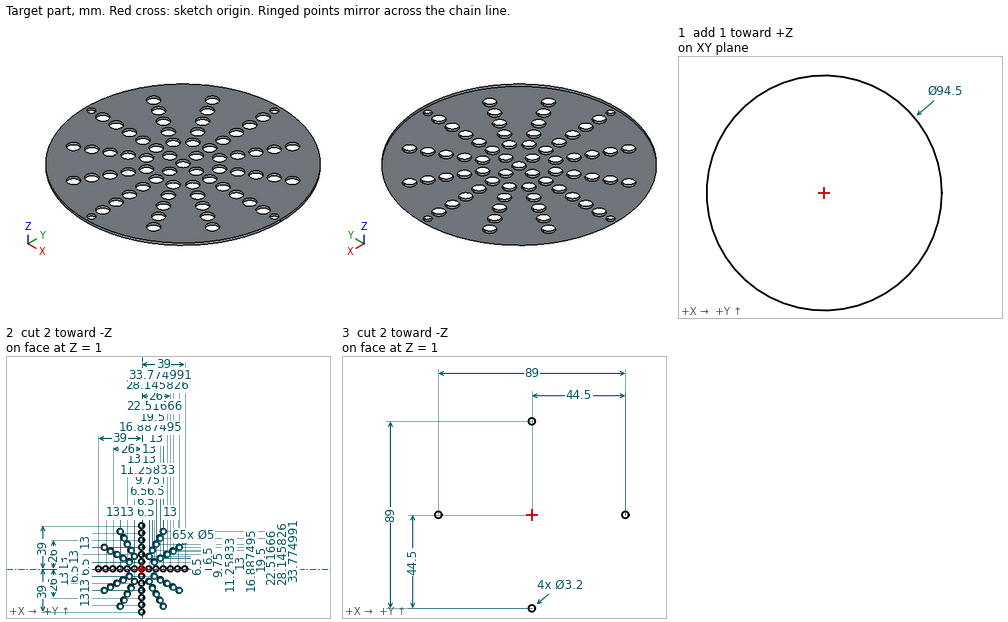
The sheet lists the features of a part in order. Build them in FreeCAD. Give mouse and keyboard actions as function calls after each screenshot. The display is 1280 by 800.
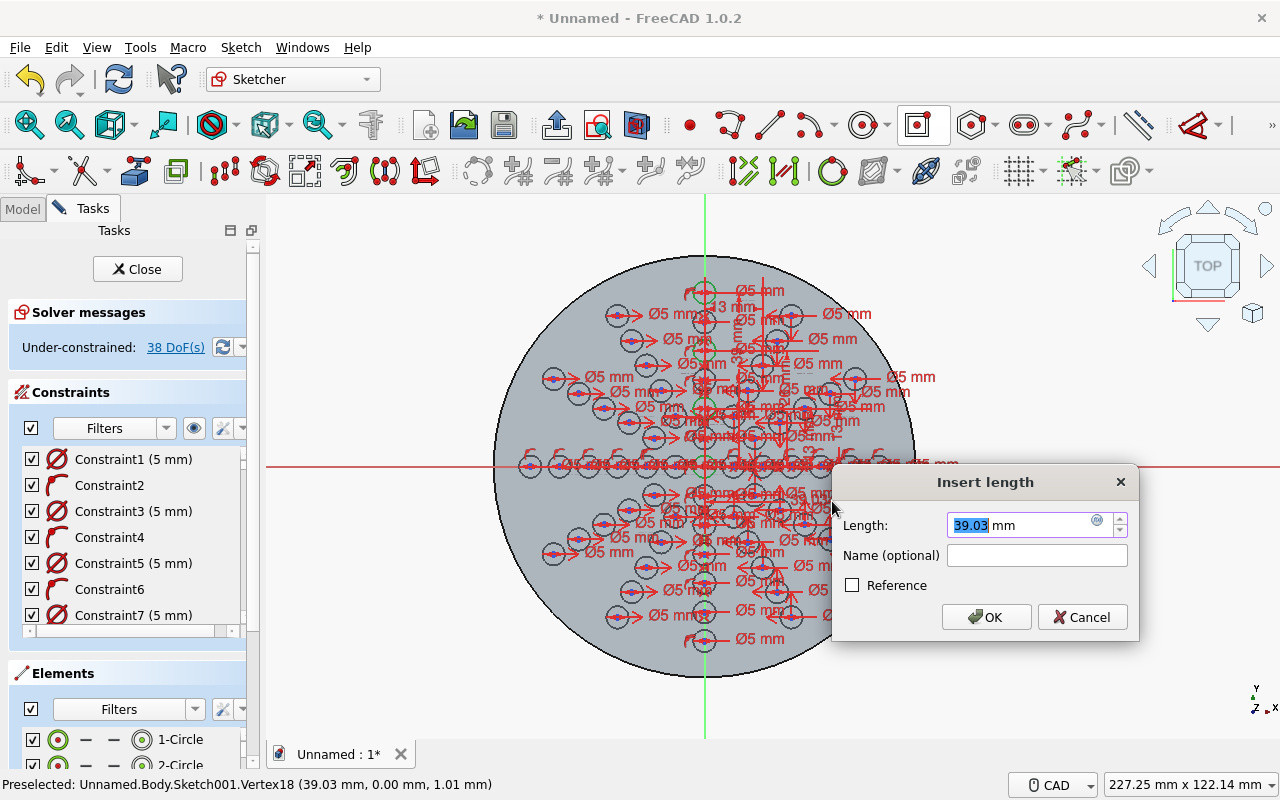
text(39)
key(Return)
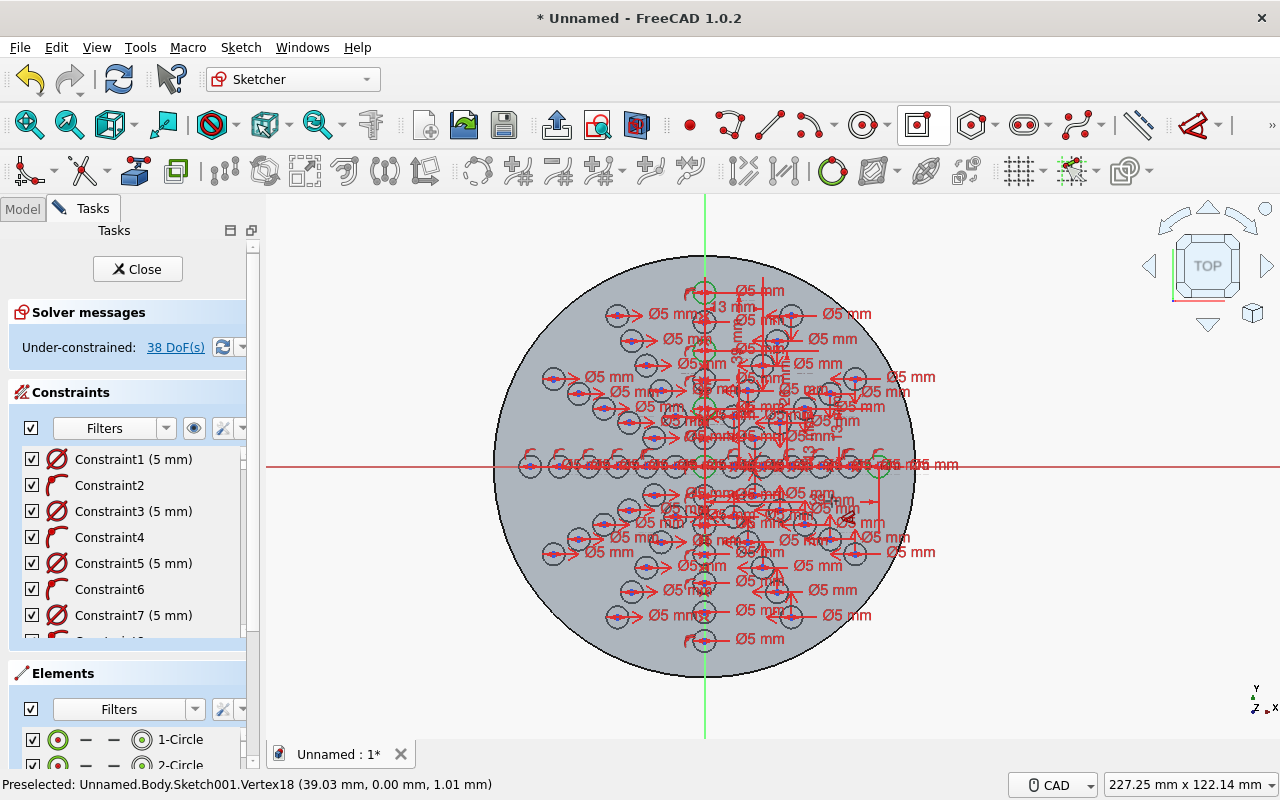
click(821, 467)
click(789, 549)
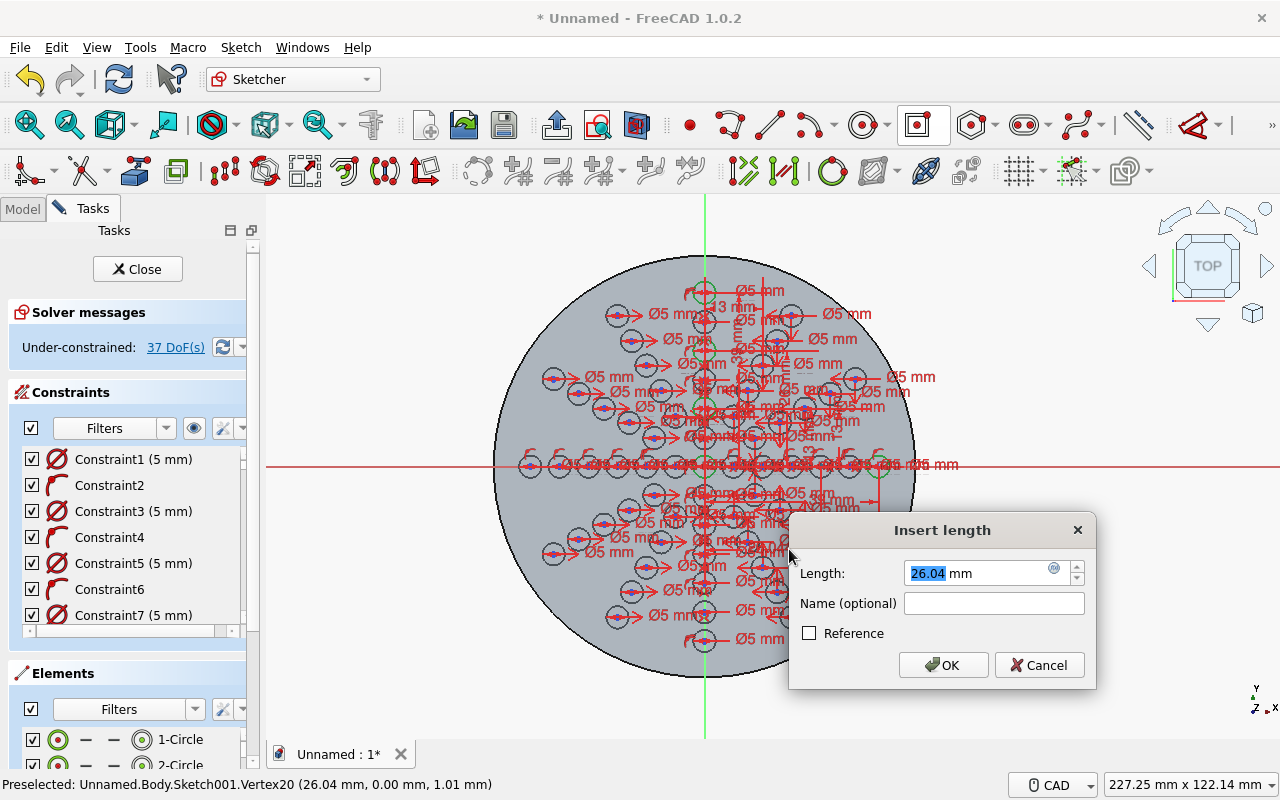
text(26)
key(Return)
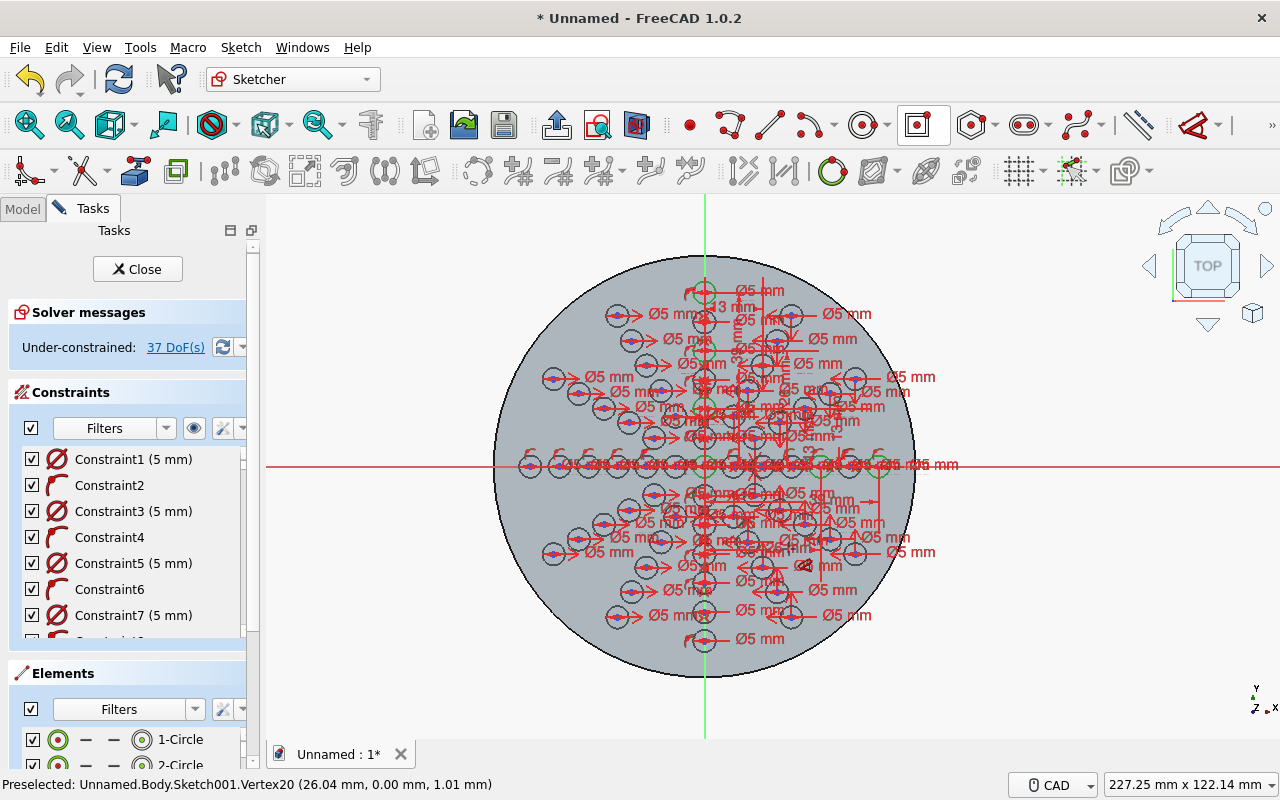
click(762, 467)
click(733, 573)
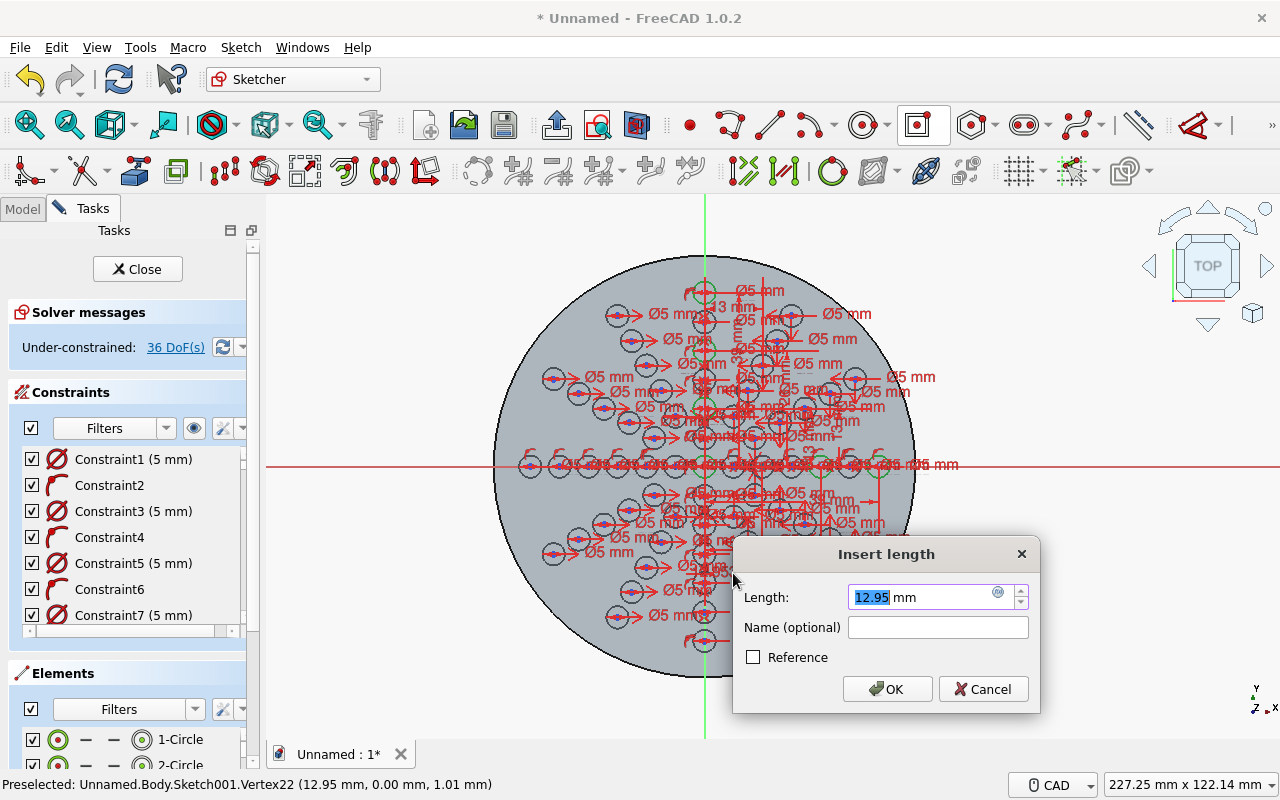
text(13)
key(Return)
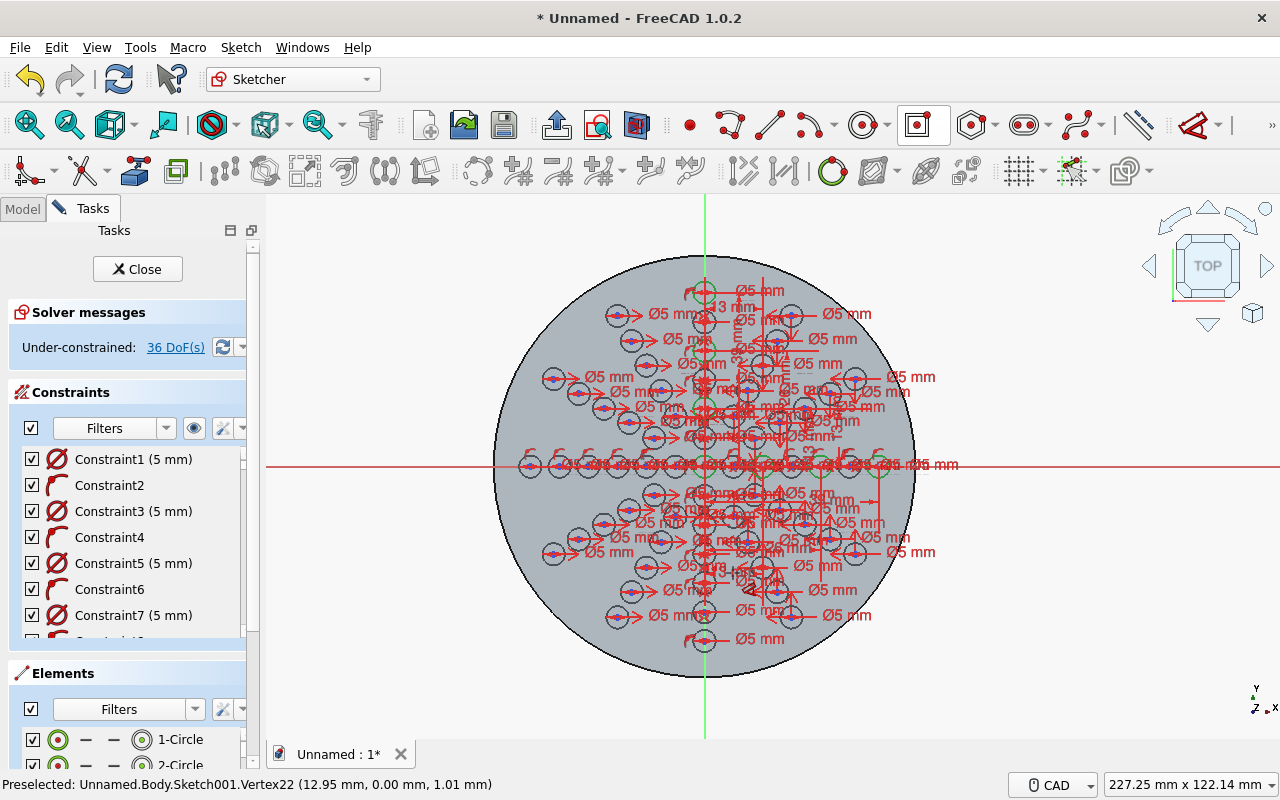
click(705, 641)
click(739, 594)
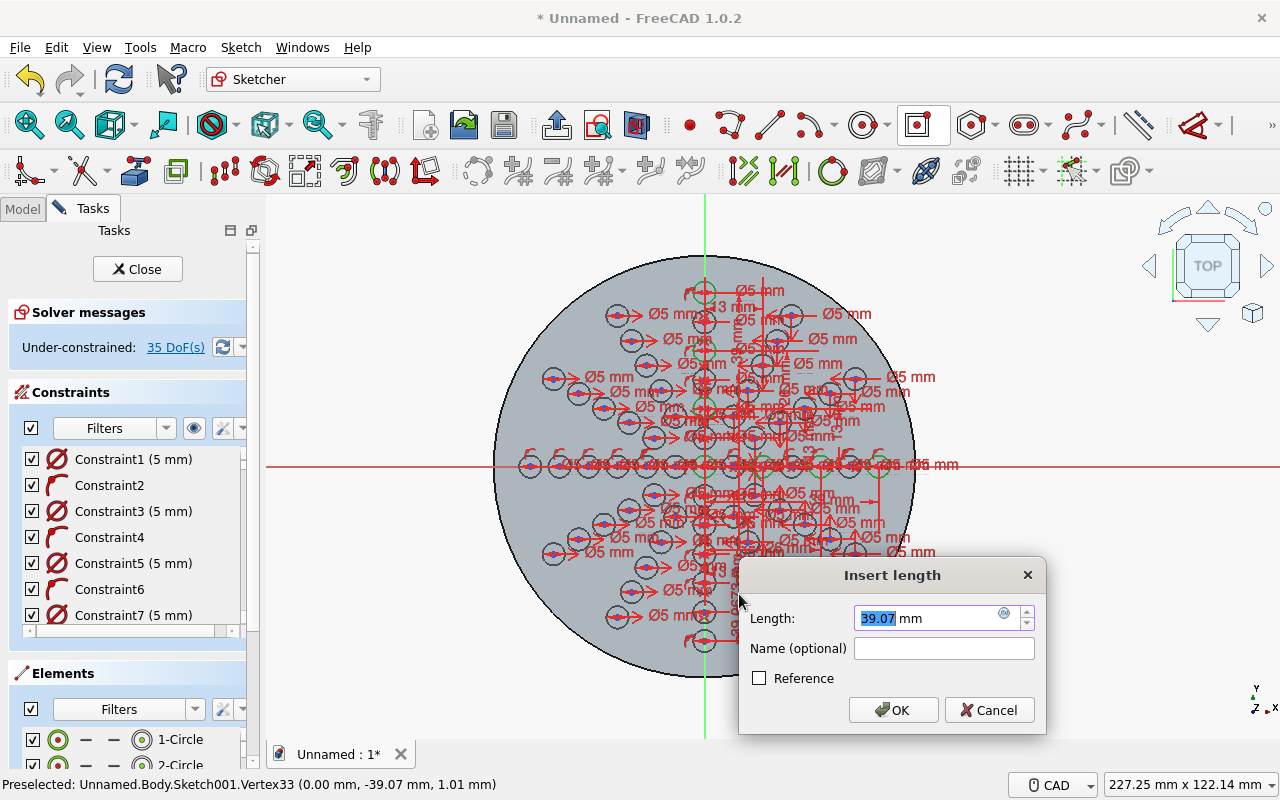
text(39)
key(Return)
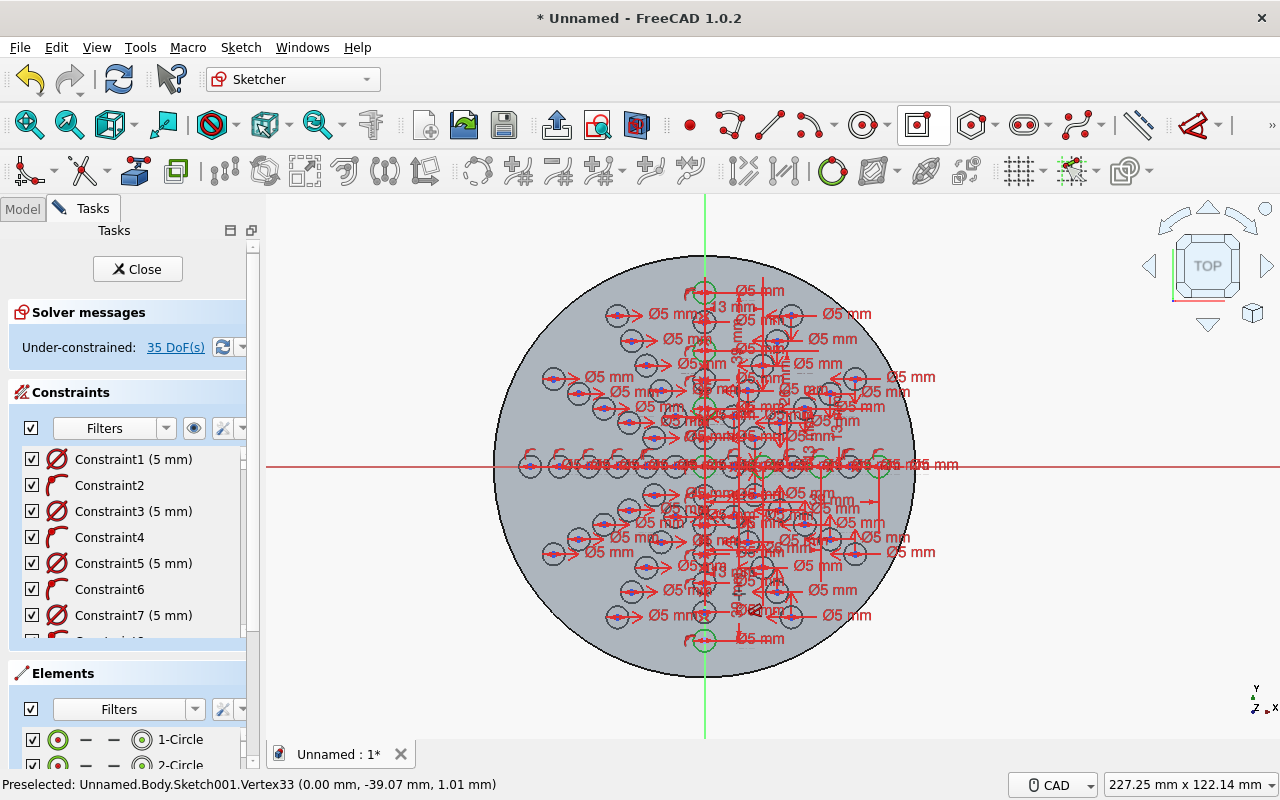
click(705, 583)
click(623, 552)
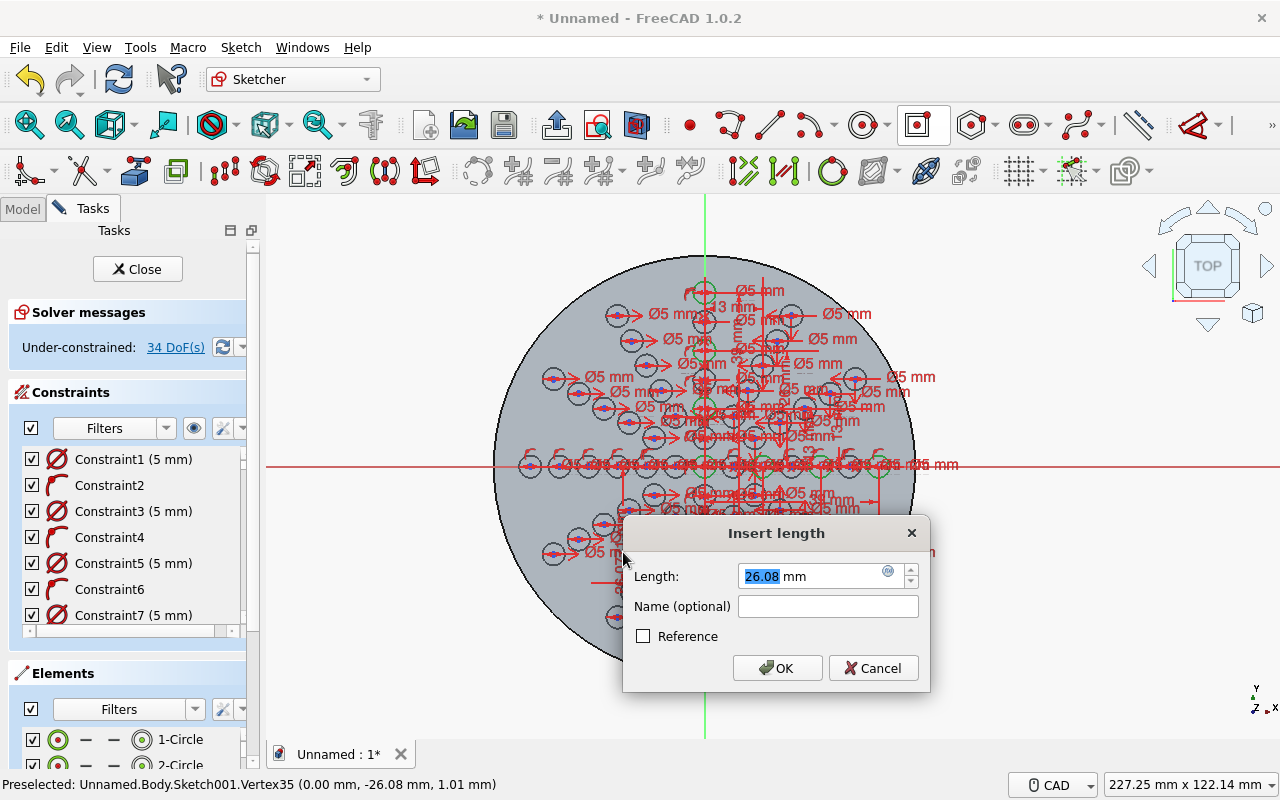
text(26)
key(Return)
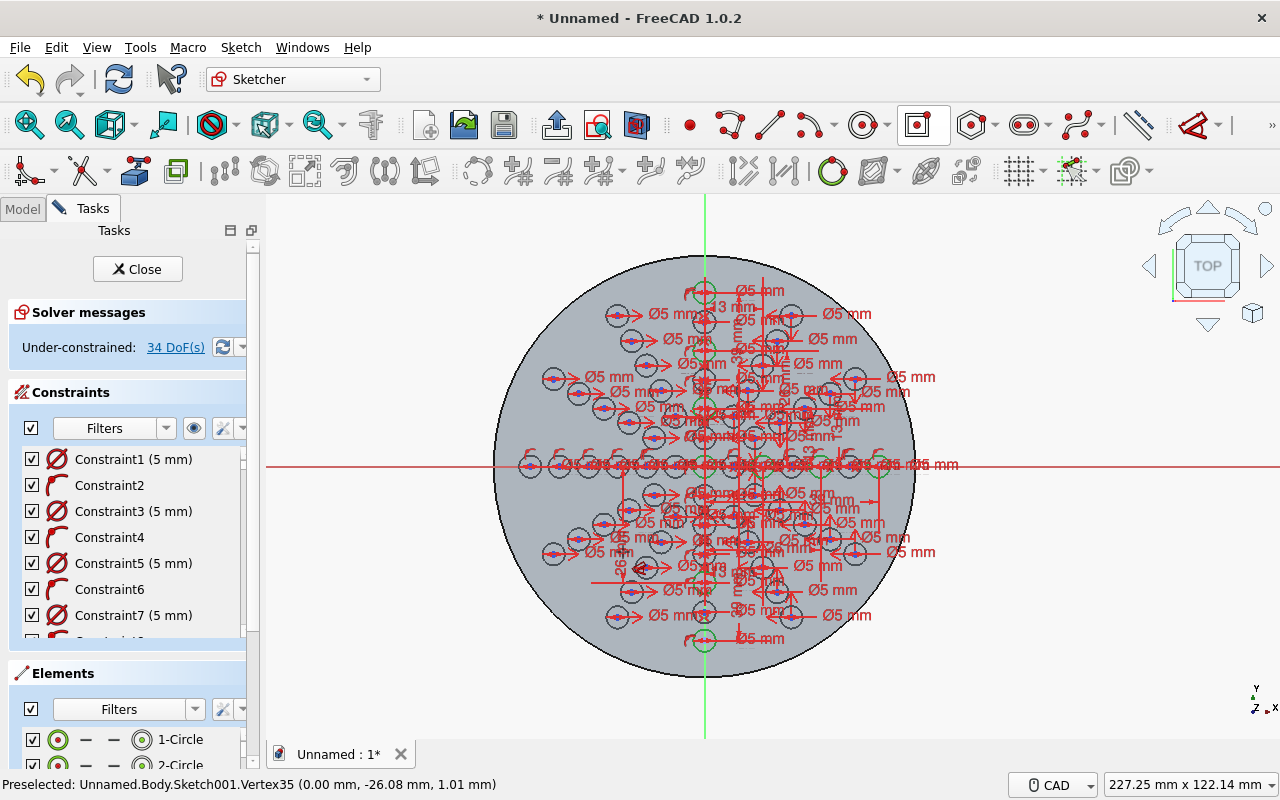
click(705, 525)
click(599, 496)